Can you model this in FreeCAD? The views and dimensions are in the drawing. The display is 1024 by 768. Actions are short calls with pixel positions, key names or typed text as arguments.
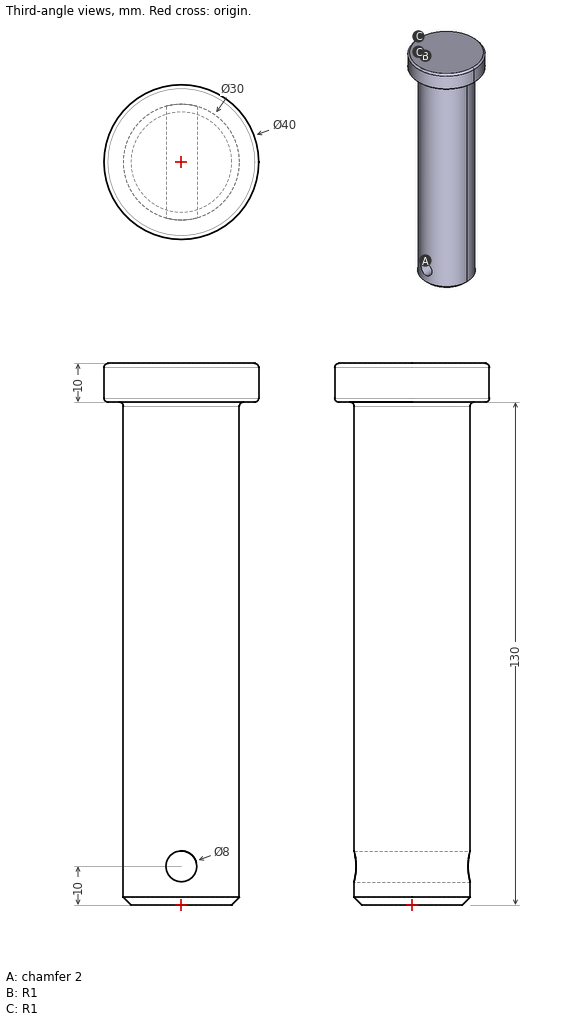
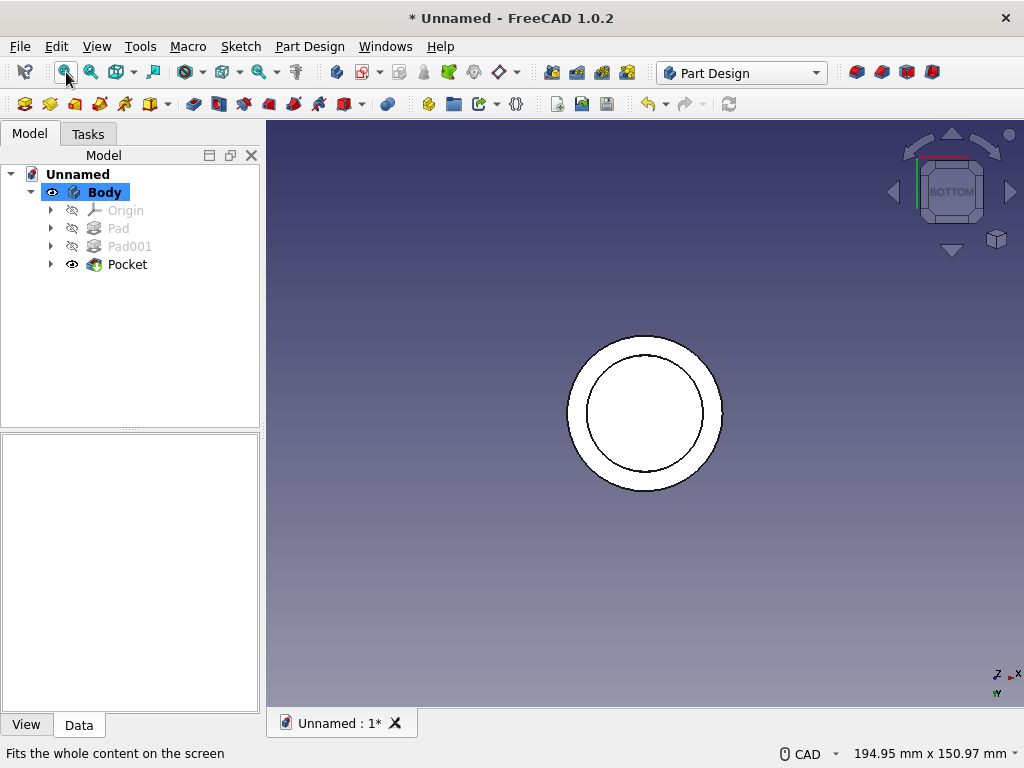
click(66, 72)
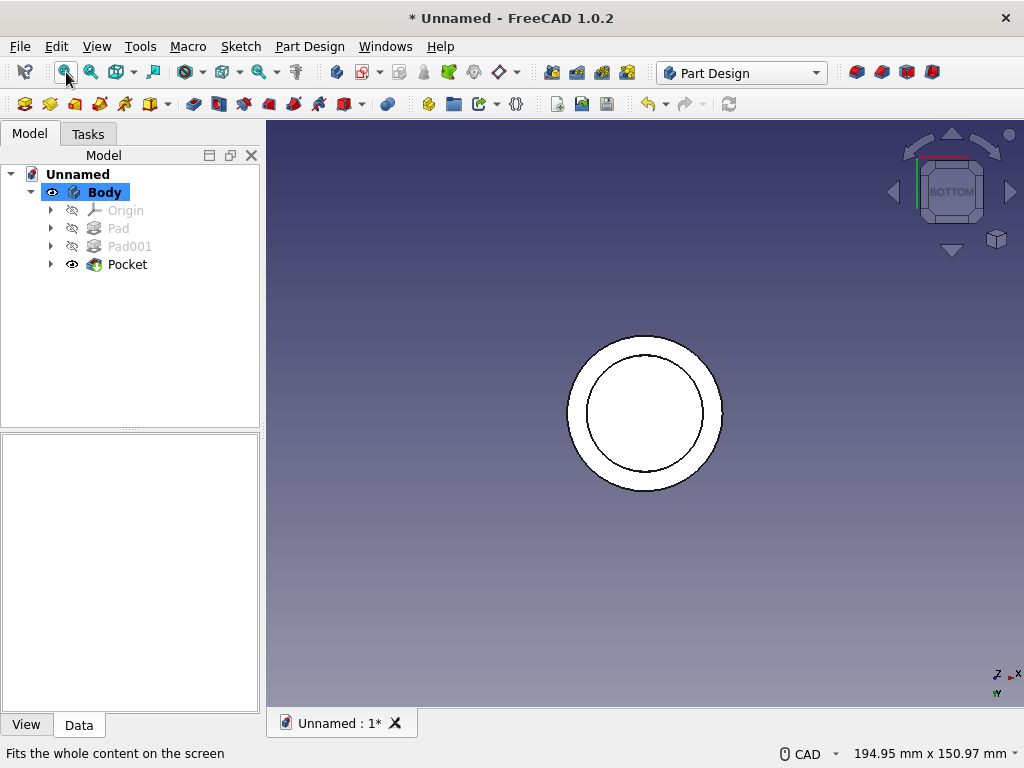
click(587, 412)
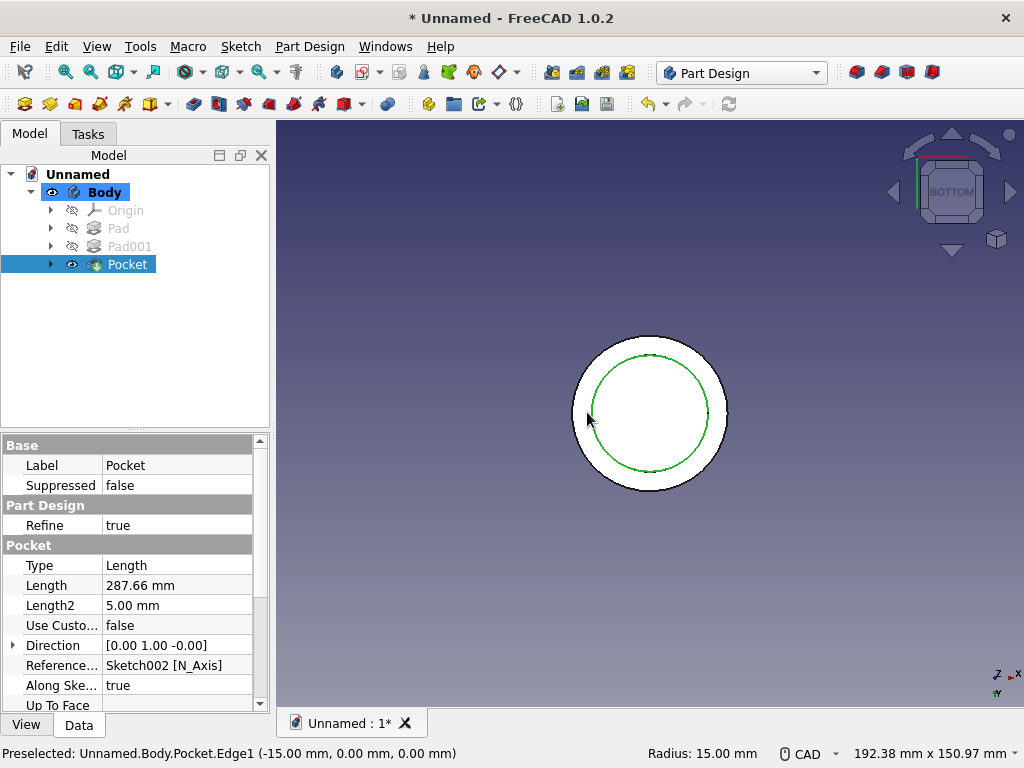
click(882, 72)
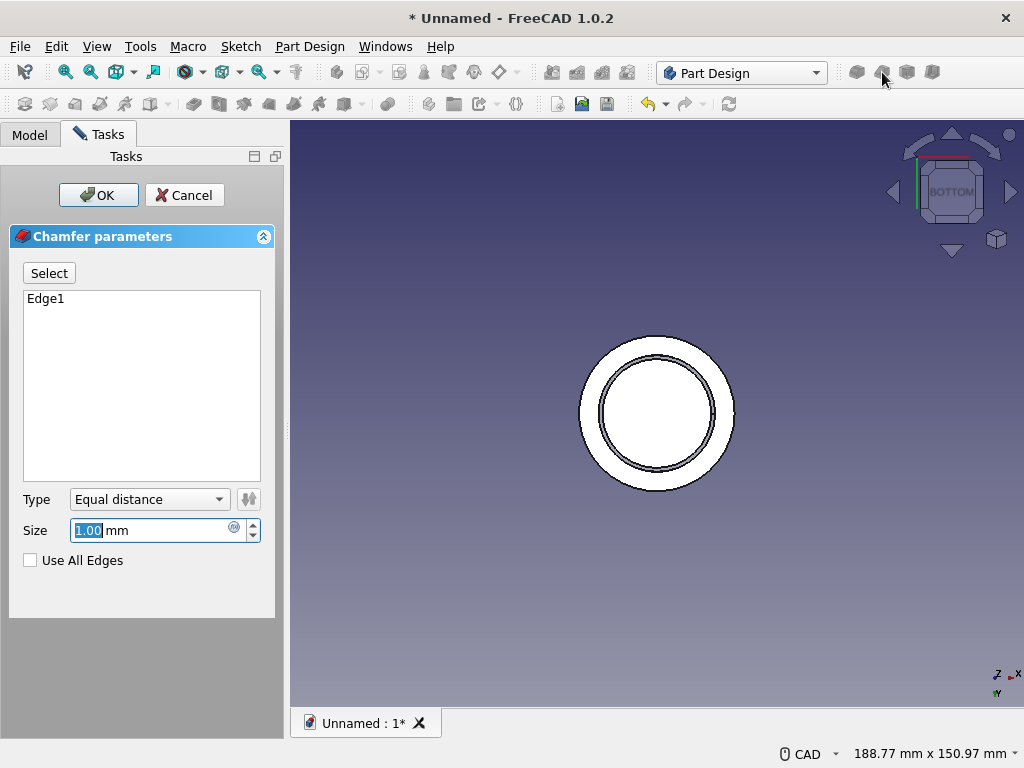
text(2)
key(Tab)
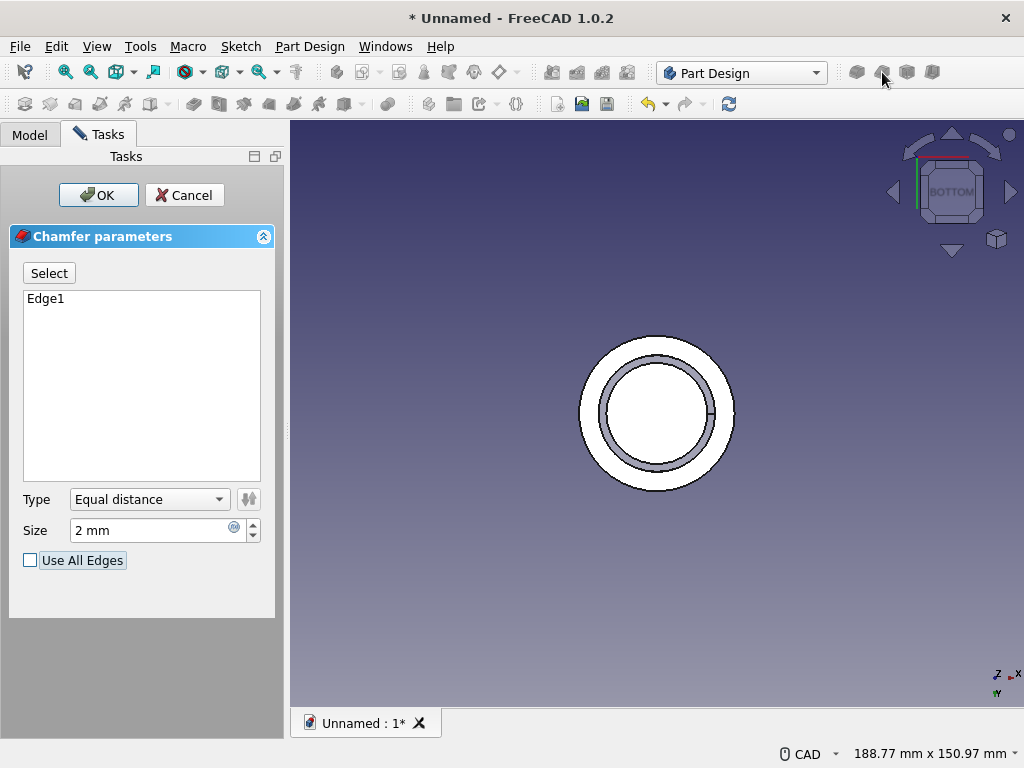
click(99, 195)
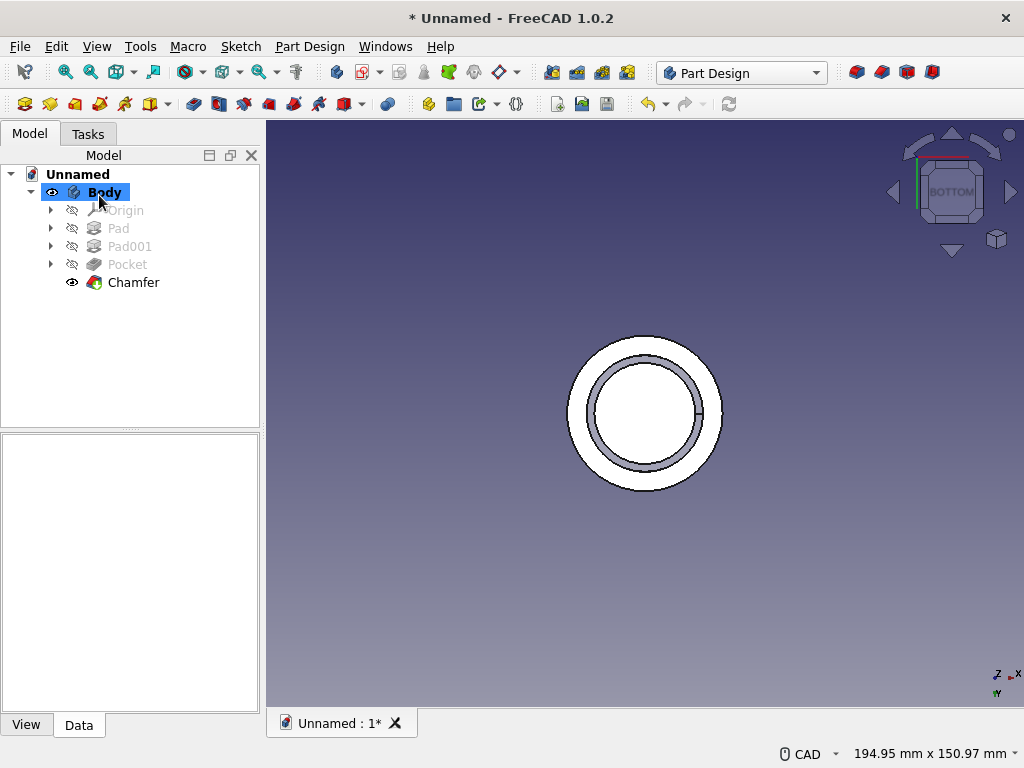
click(66, 72)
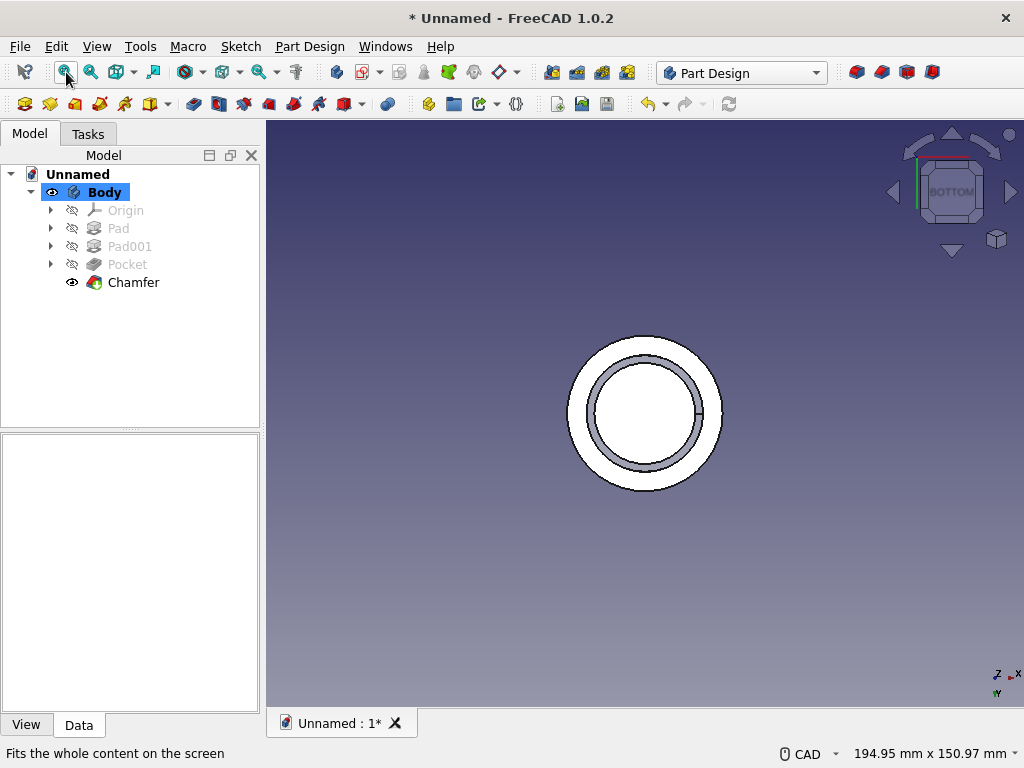
key(0)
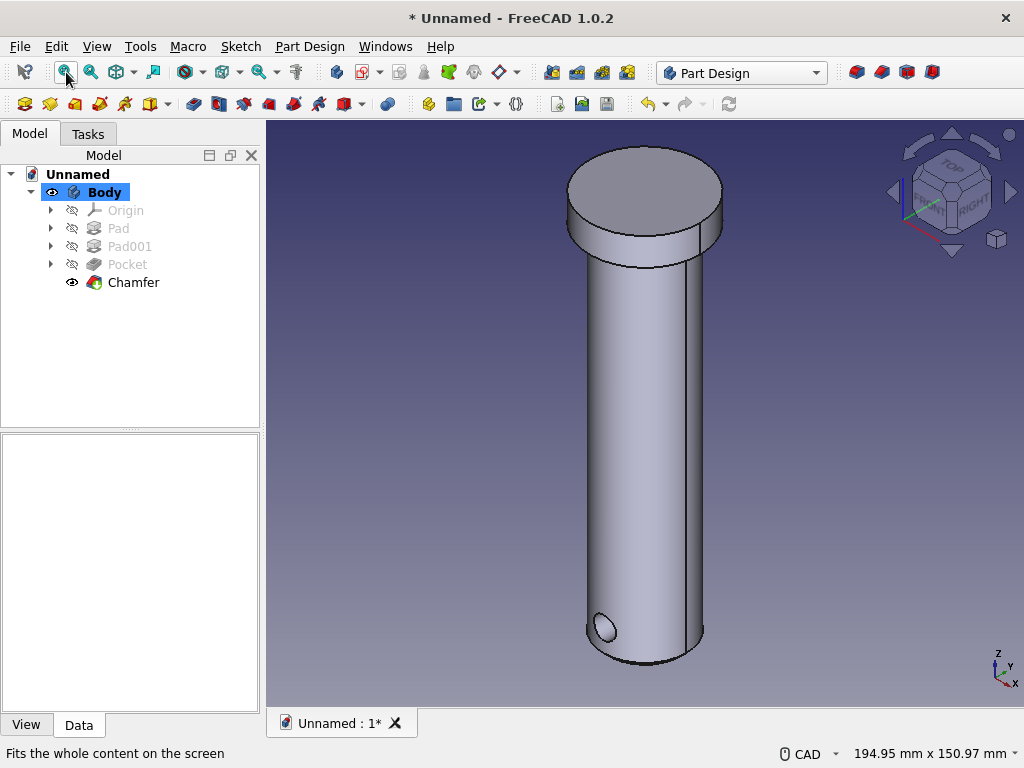
key(2)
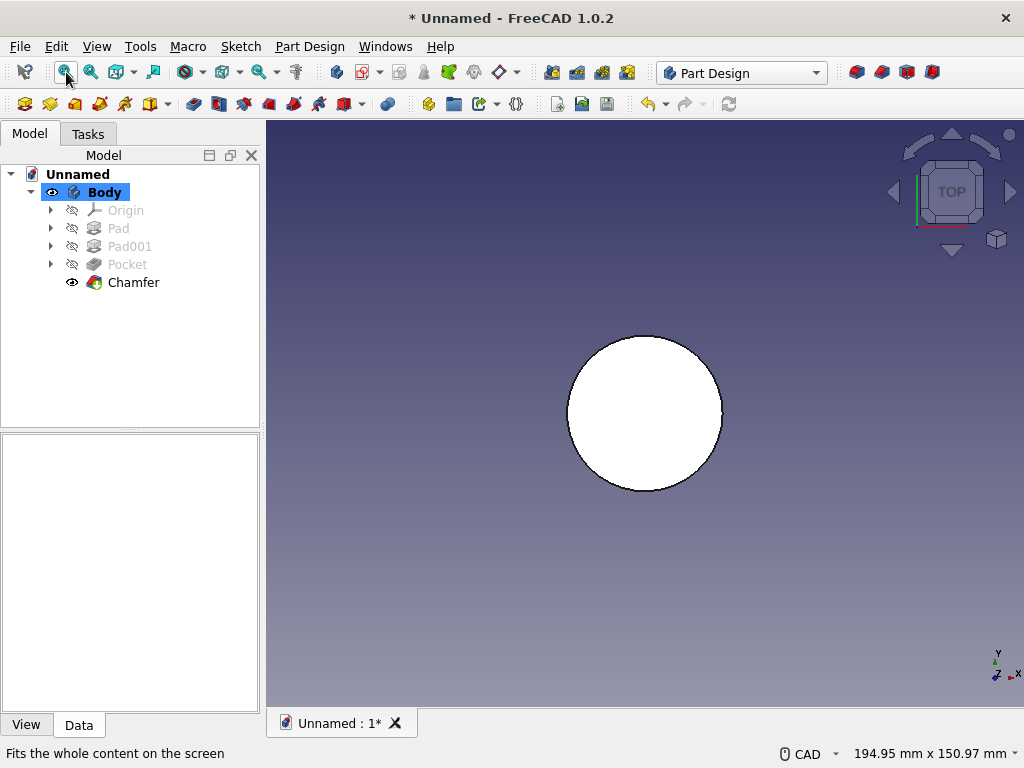
click(66, 72)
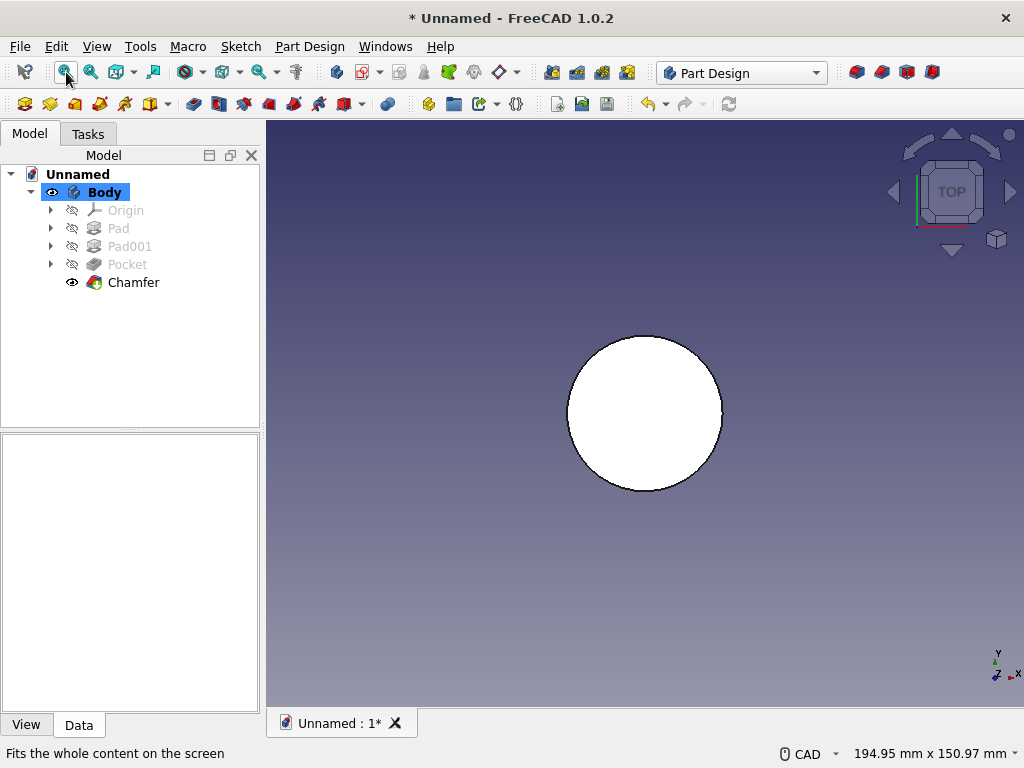
key(1)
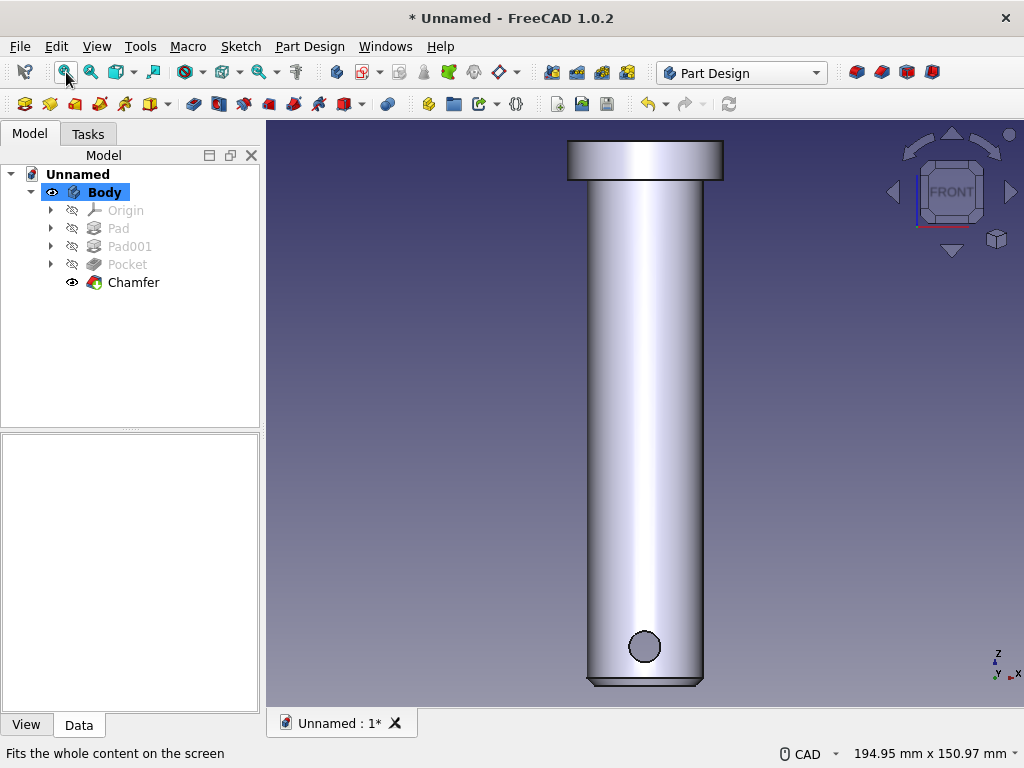
key(3)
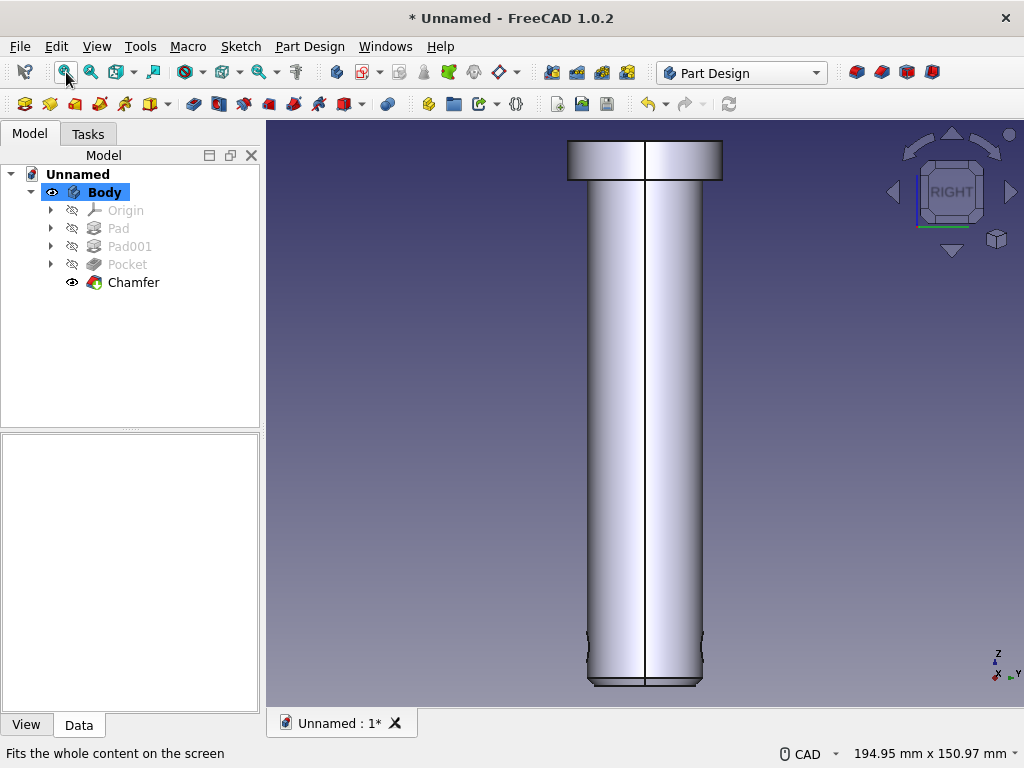
key(5)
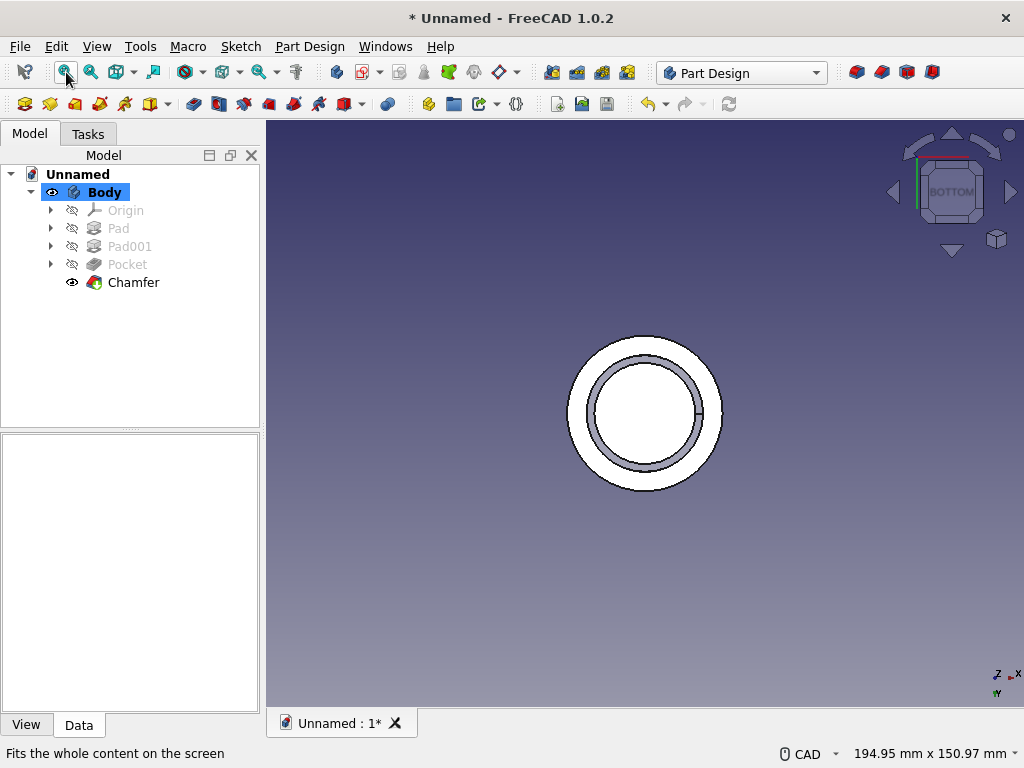
click(66, 72)